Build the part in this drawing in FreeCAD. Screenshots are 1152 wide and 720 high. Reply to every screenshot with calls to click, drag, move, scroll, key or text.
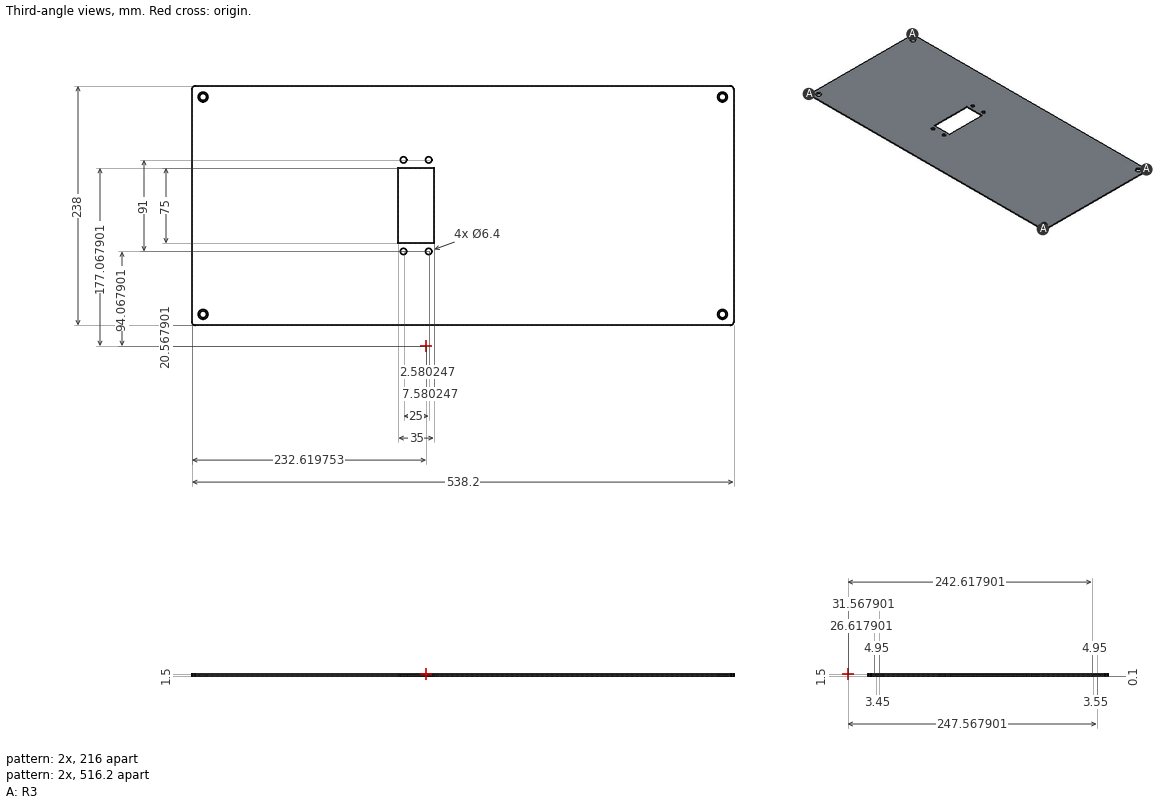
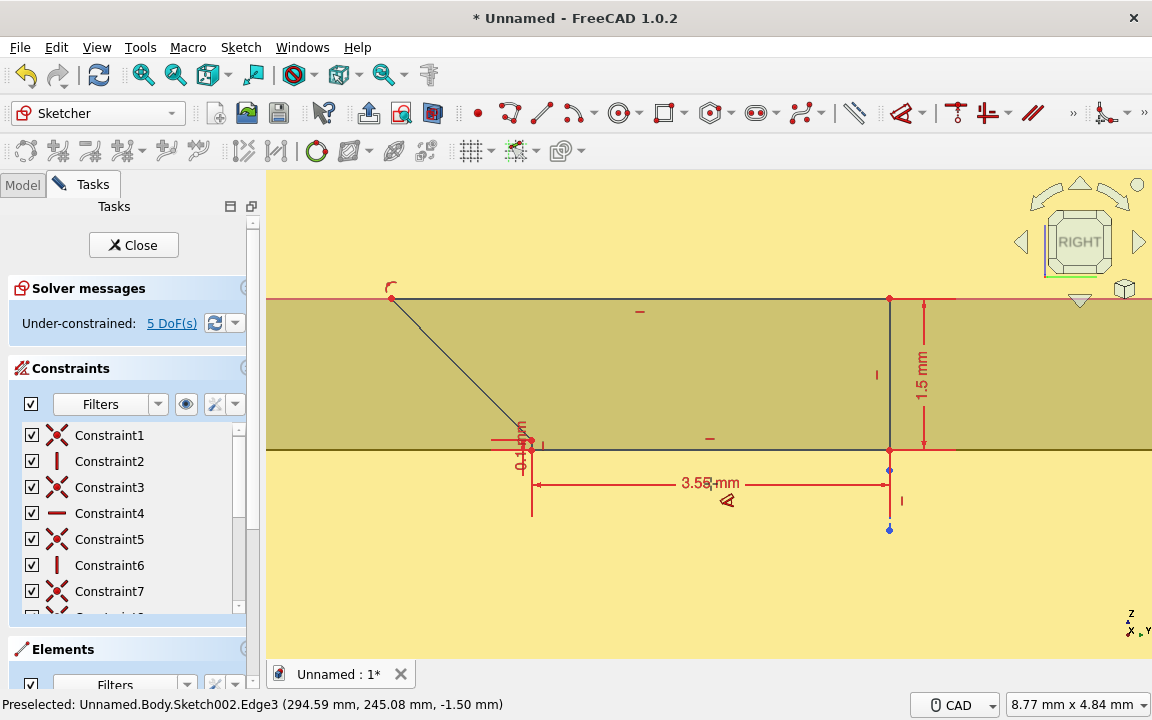
click(740, 299)
click(641, 265)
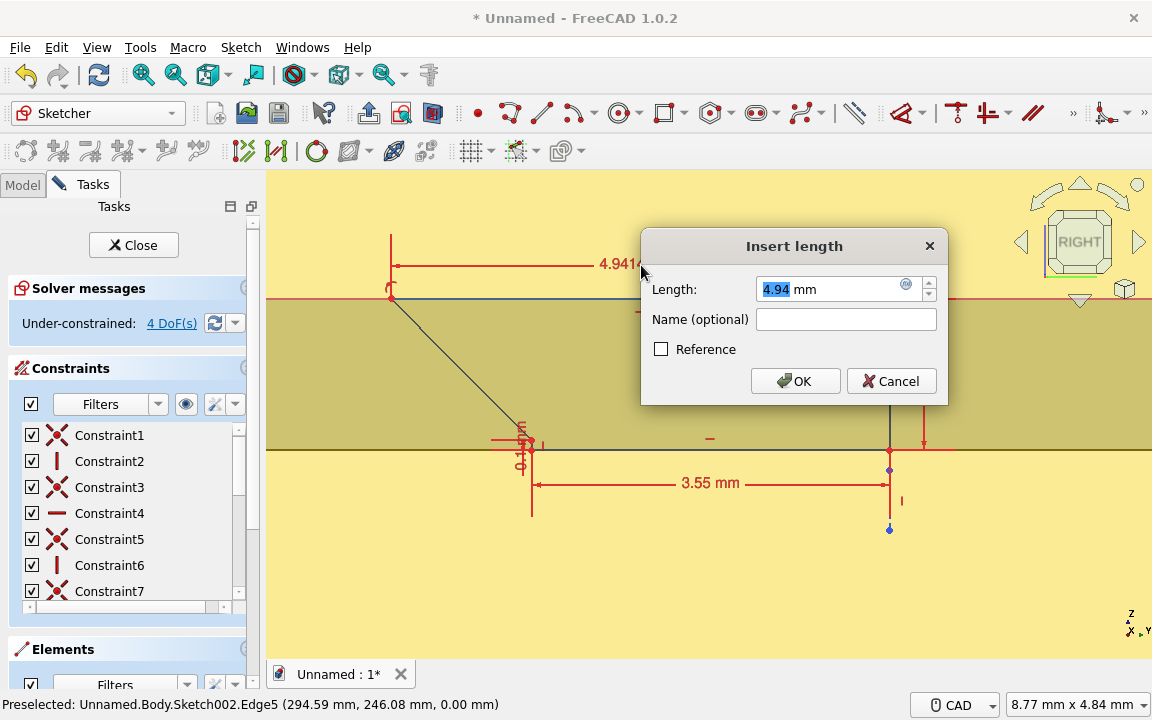
text(4.95)
key(Return)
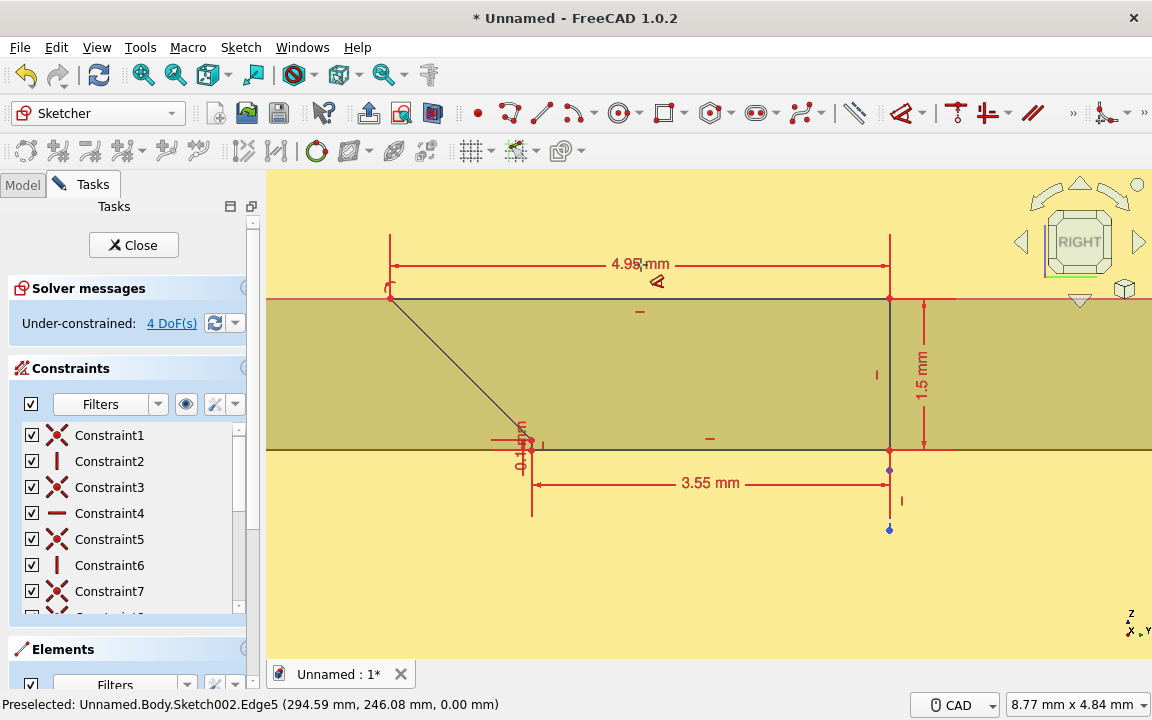
click(390, 299)
click(342, 265)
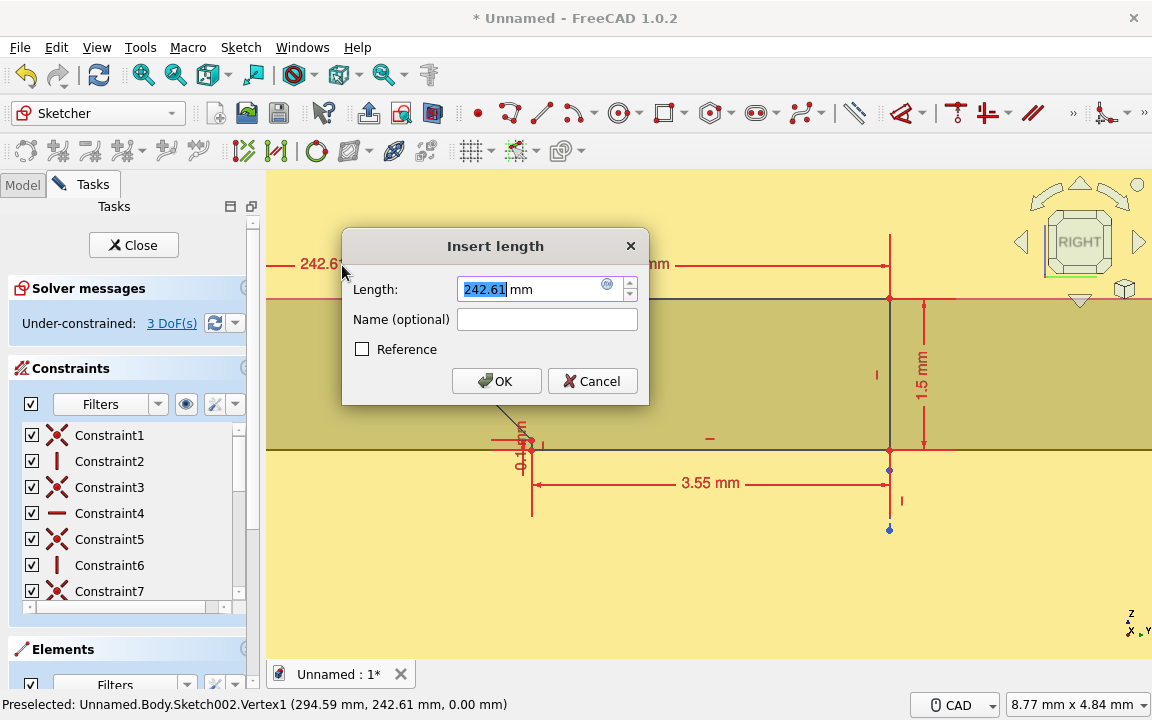
text(242.617901)
key(Return)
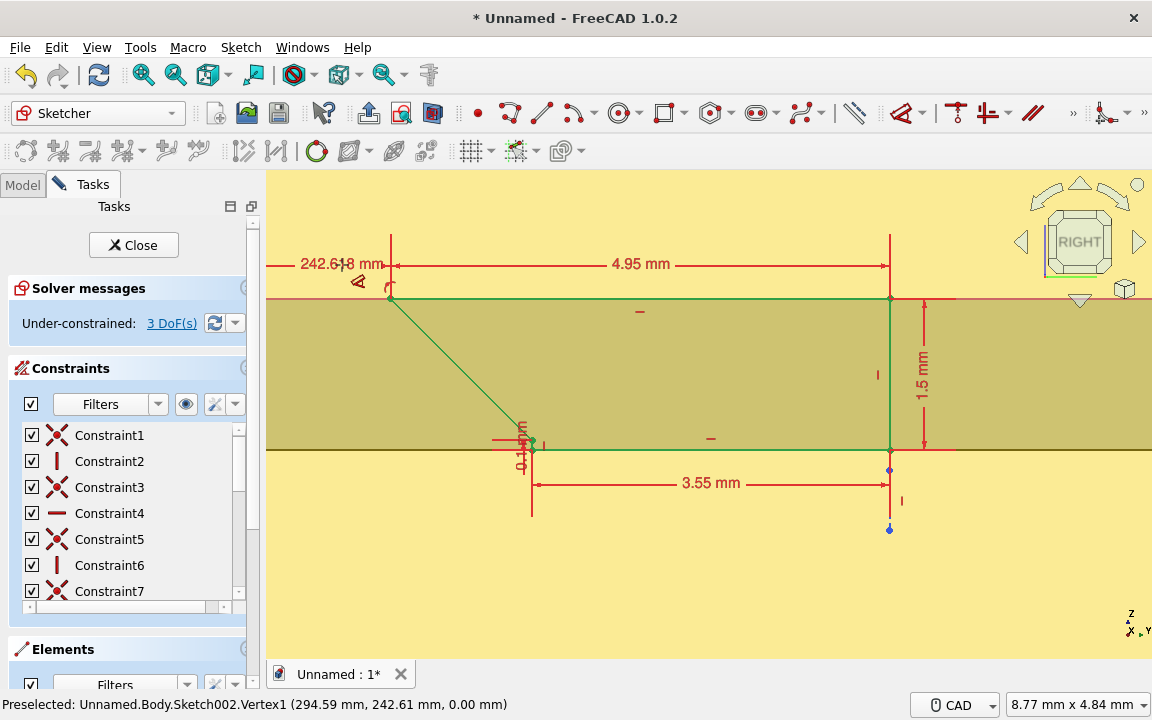
click(890, 471)
click(455, 265)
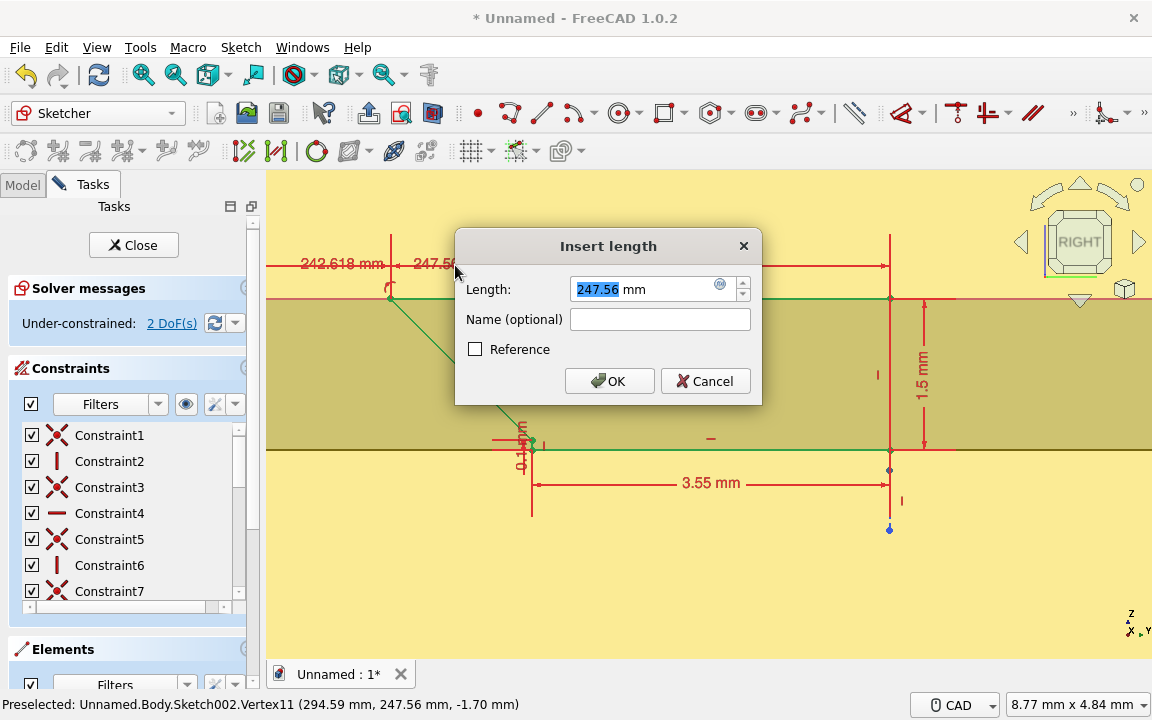
text(247.567901)
key(Return)
key(Escape)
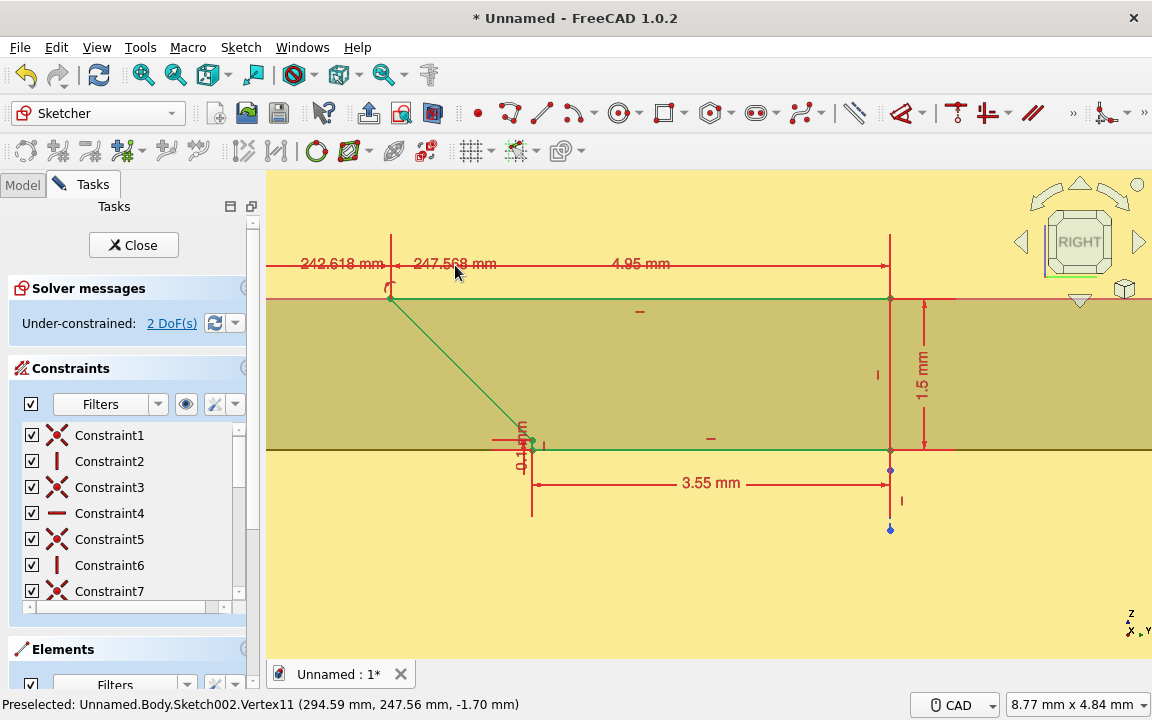
click(134, 245)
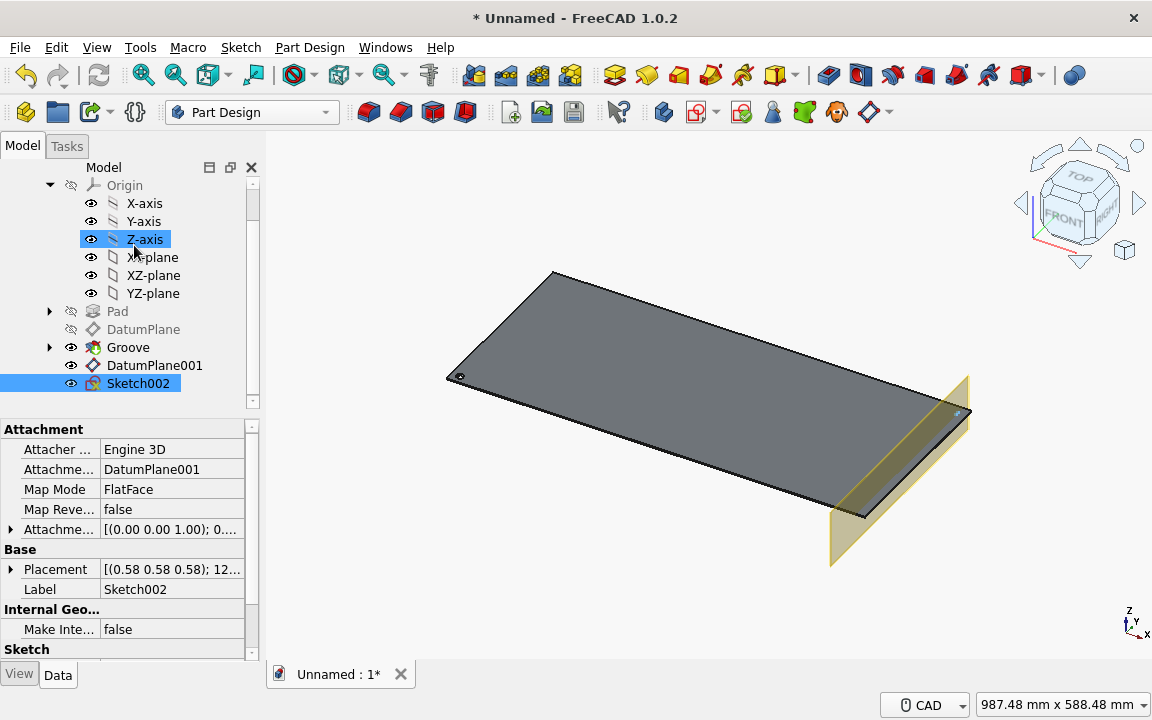
click(894, 76)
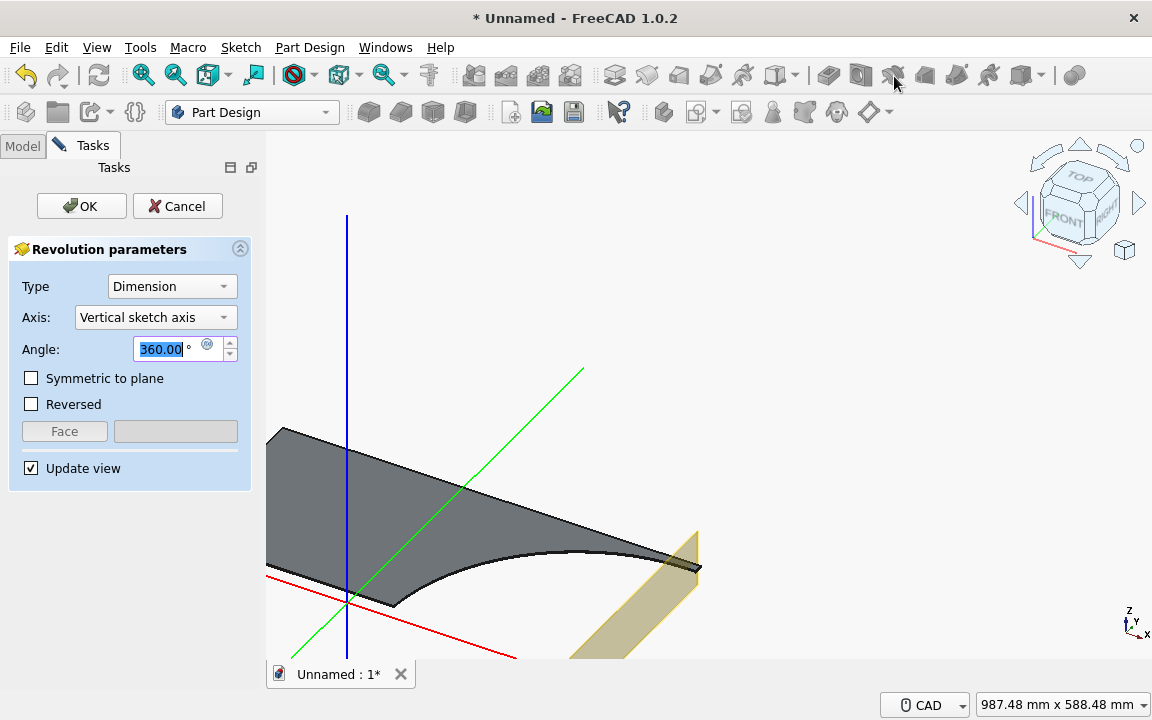
click(156, 318)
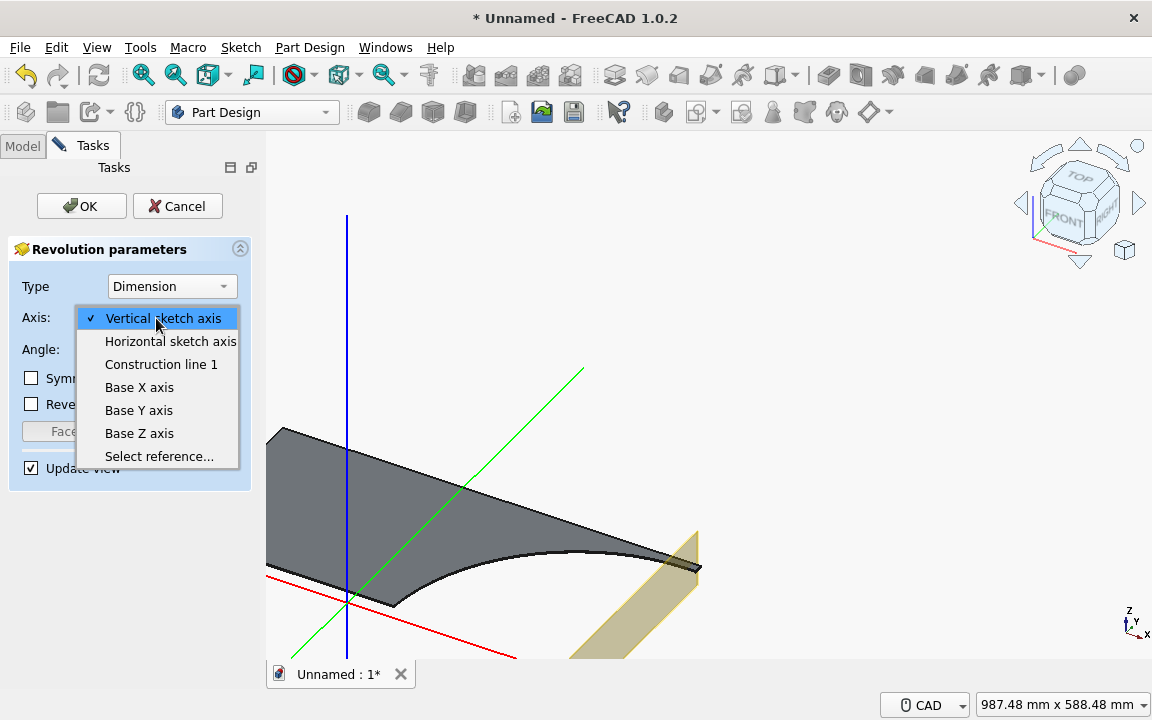
click(156, 364)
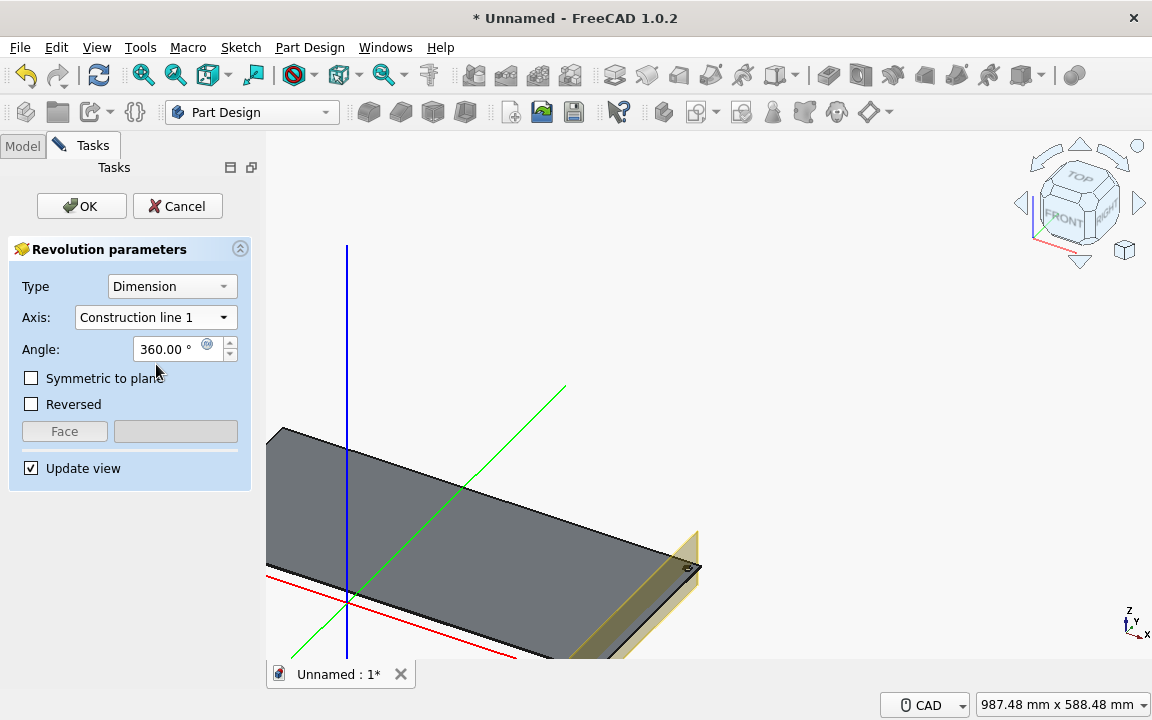
click(82, 206)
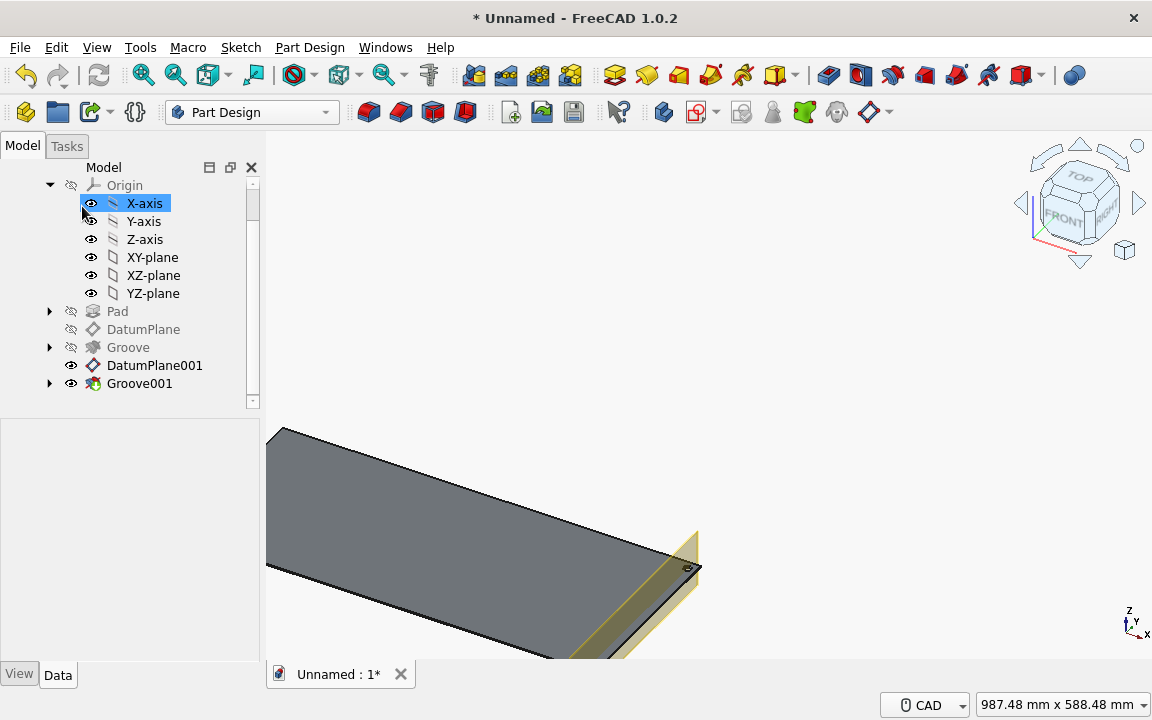
click(116, 365)
key(space)